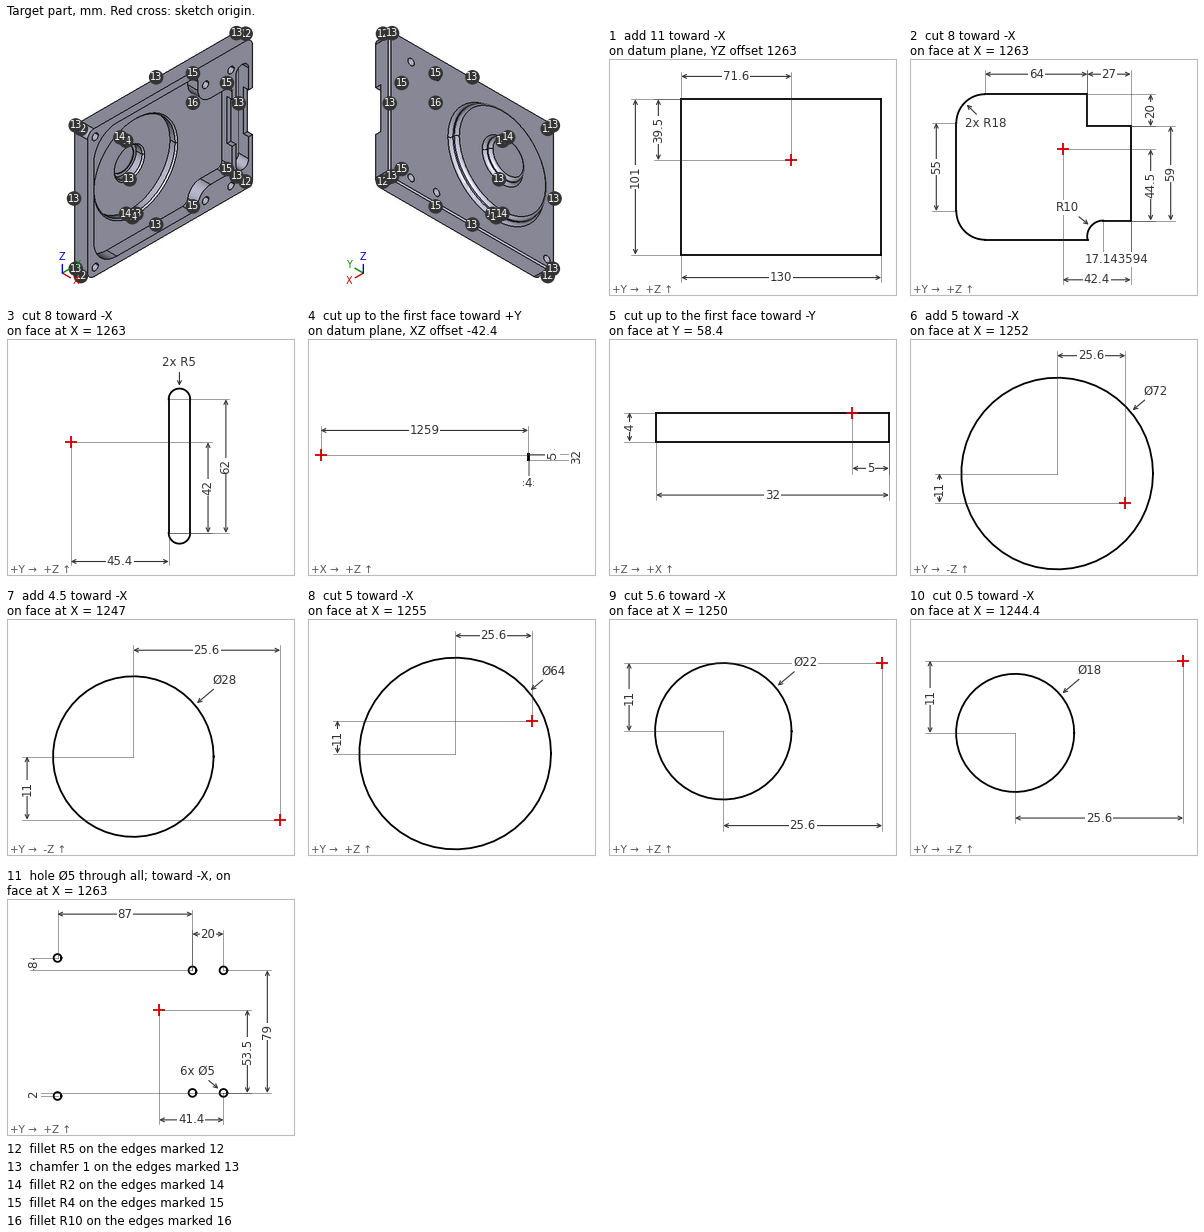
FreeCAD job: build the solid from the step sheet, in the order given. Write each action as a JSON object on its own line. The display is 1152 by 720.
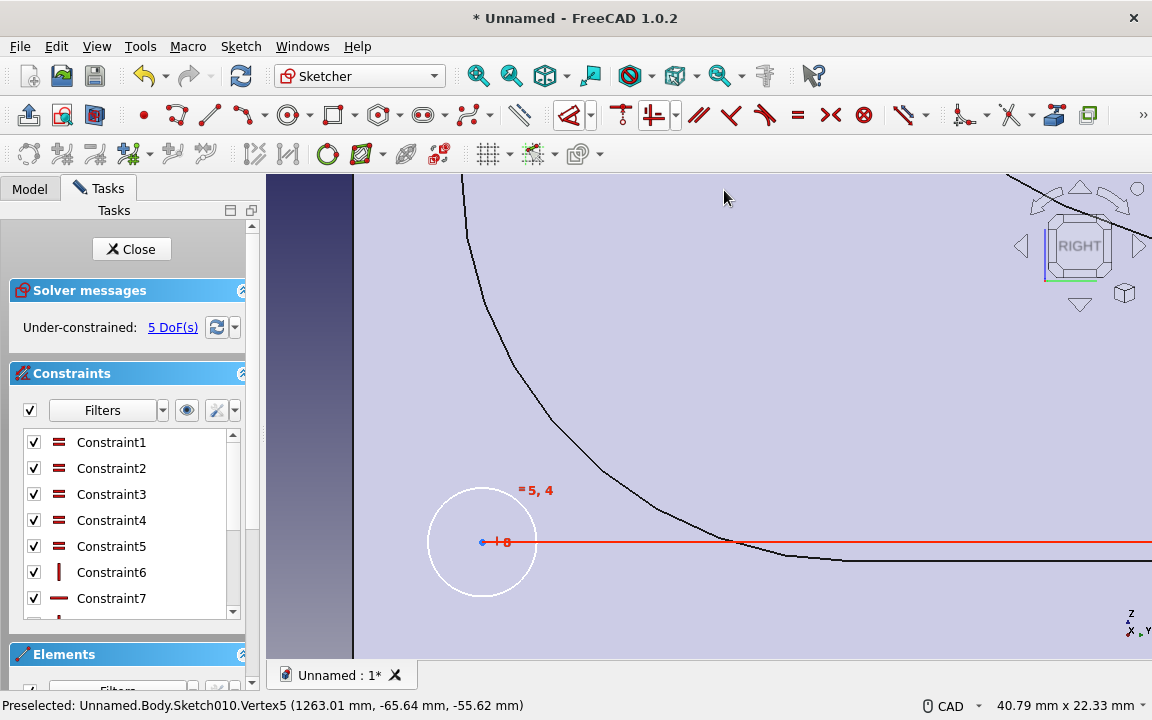
{"action": "scroll", "coordinate": [483, 549], "scroll_direction": "down", "scroll_amount": 10}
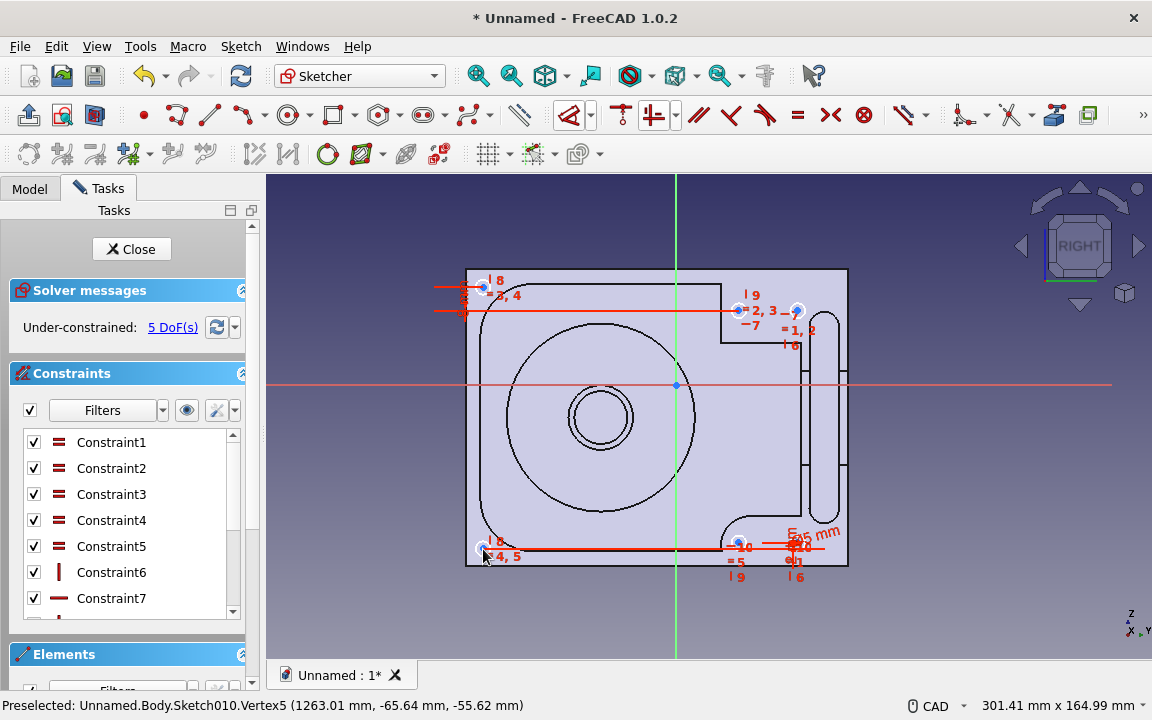
{"action": "left_click", "coordinate": [798, 543]}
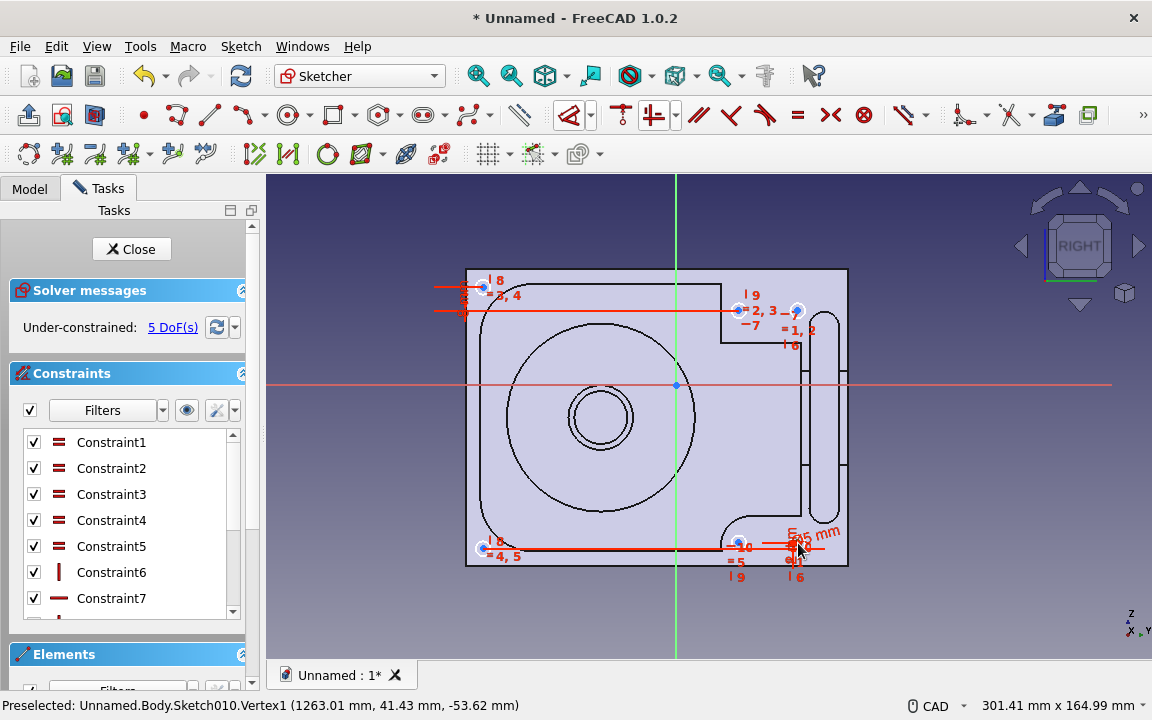
{"action": "left_click", "coordinate": [798, 311]}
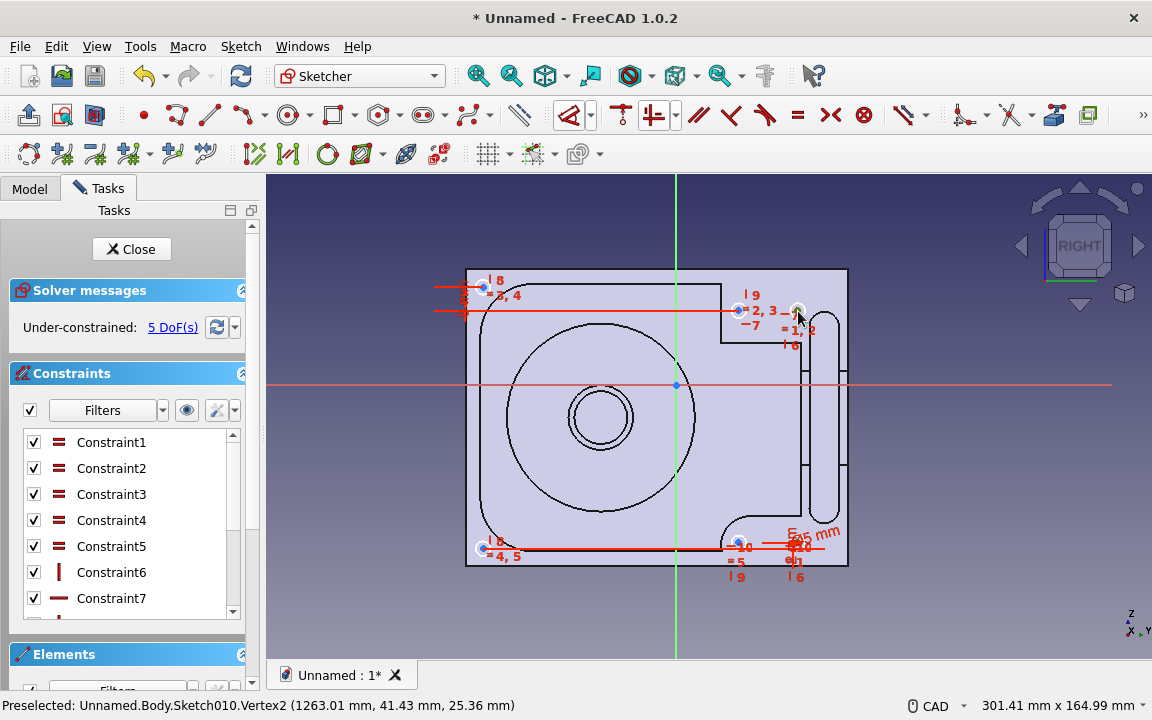
{"action": "key", "text": "i"}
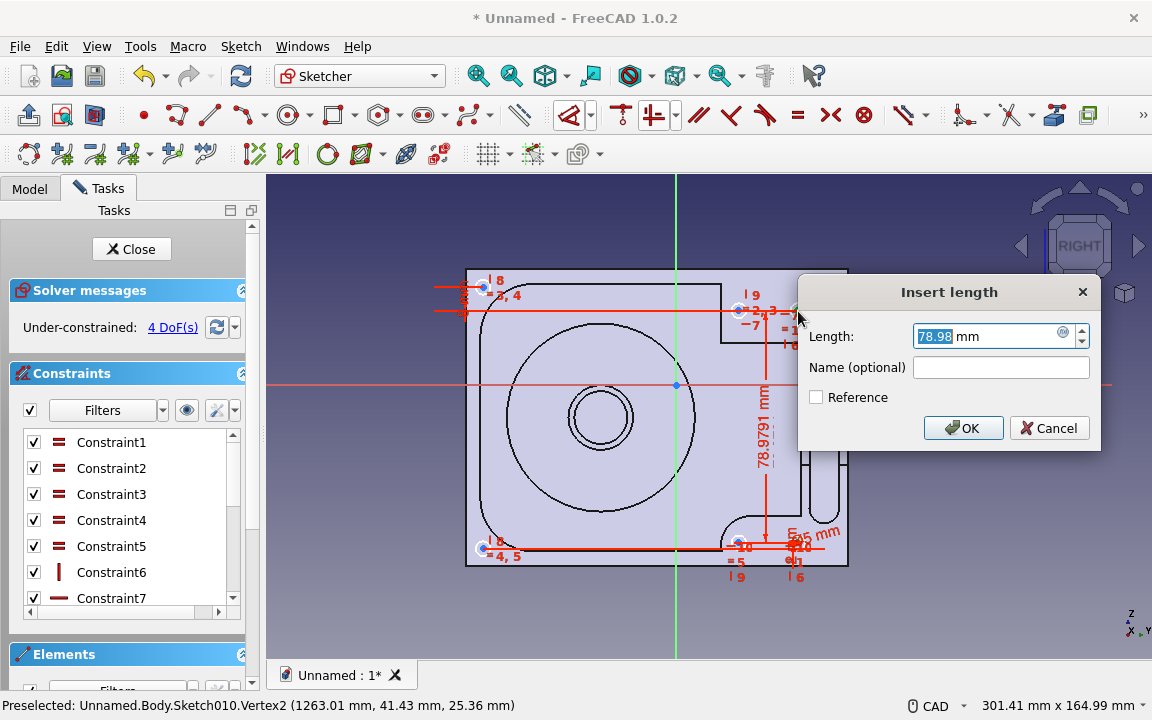
{"action": "type", "text": "79"}
{"action": "key", "text": "Return"}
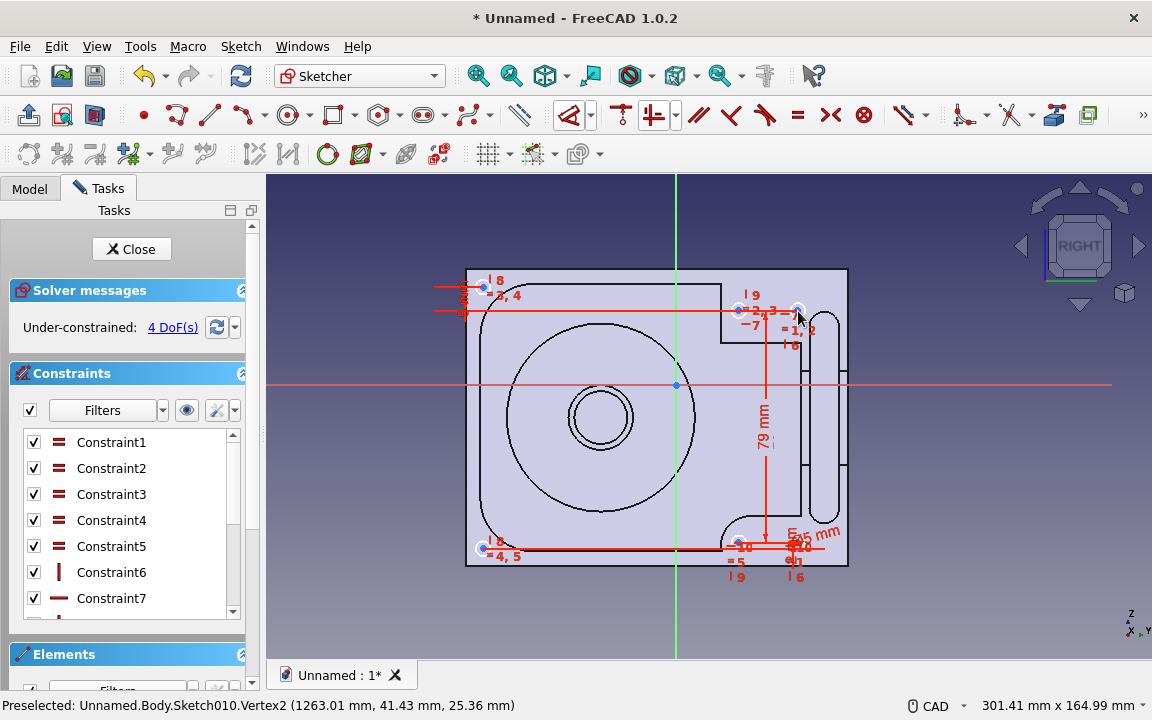
{"action": "left_click", "coordinate": [798, 311]}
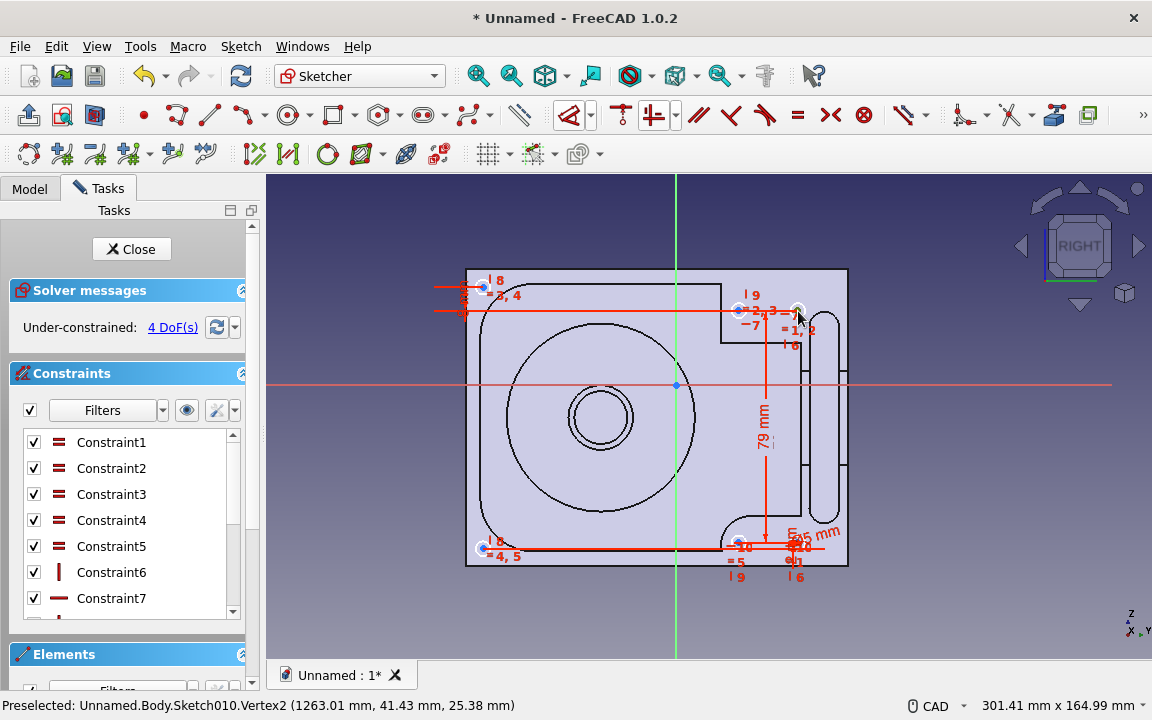
{"action": "left_click", "coordinate": [739, 311]}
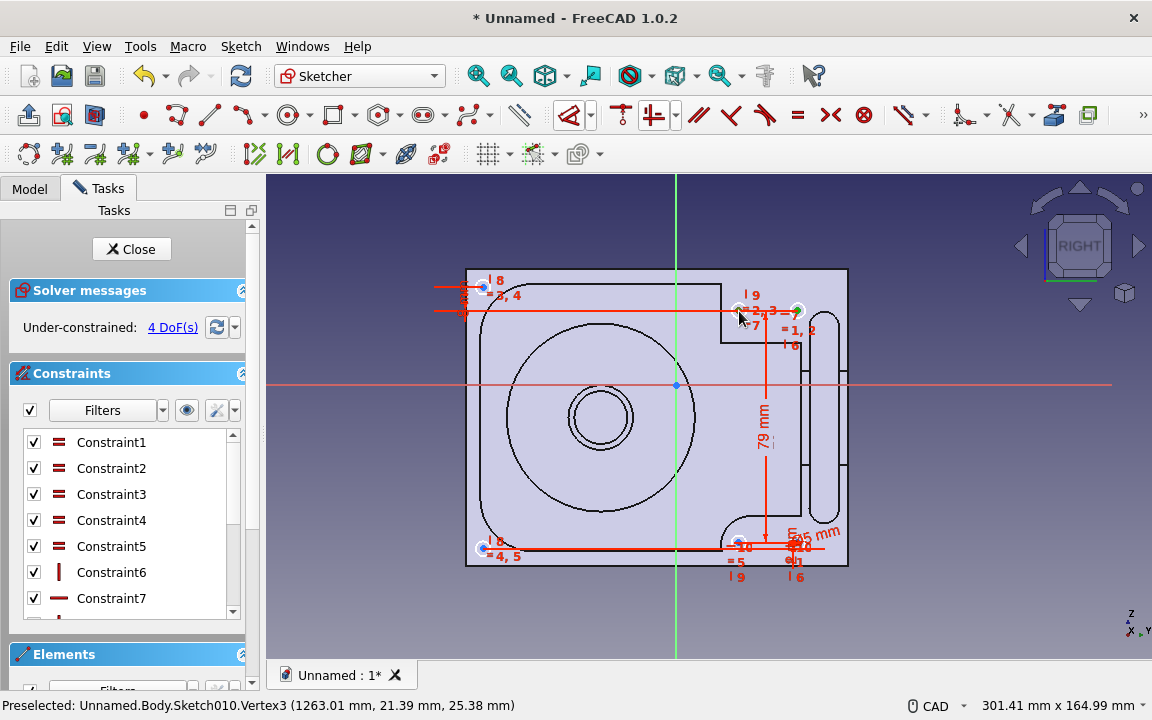
{"action": "left_click", "coordinate": [590, 116]}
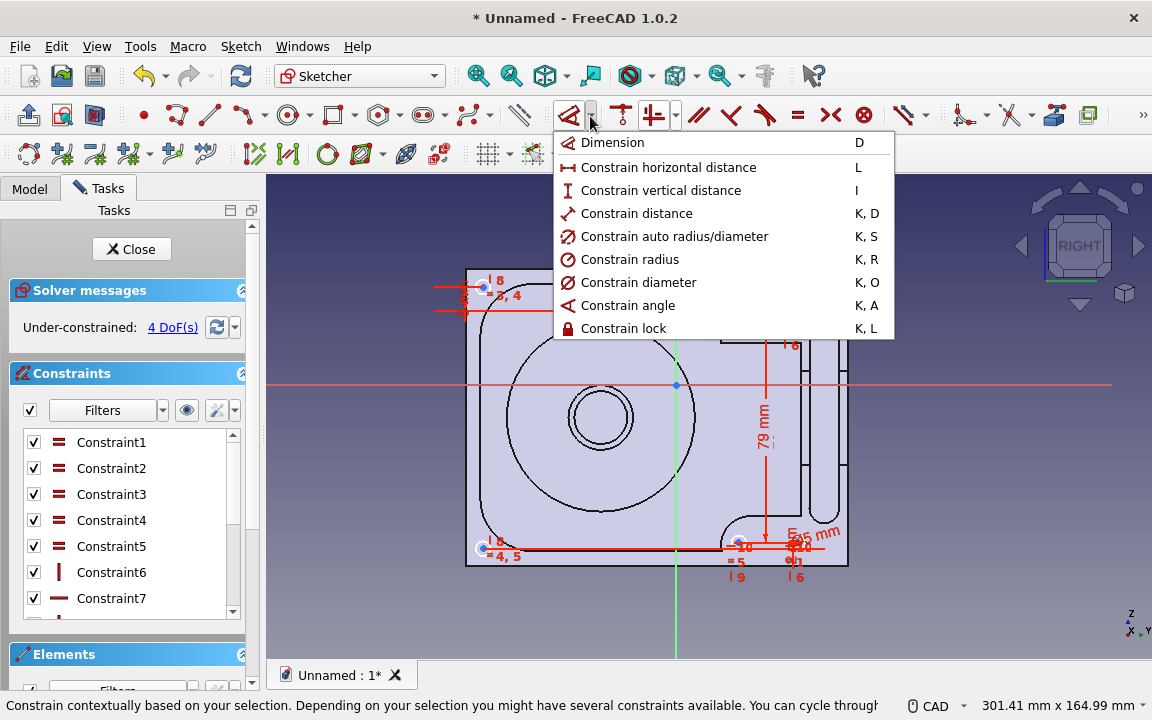
{"action": "left_click", "coordinate": [724, 168]}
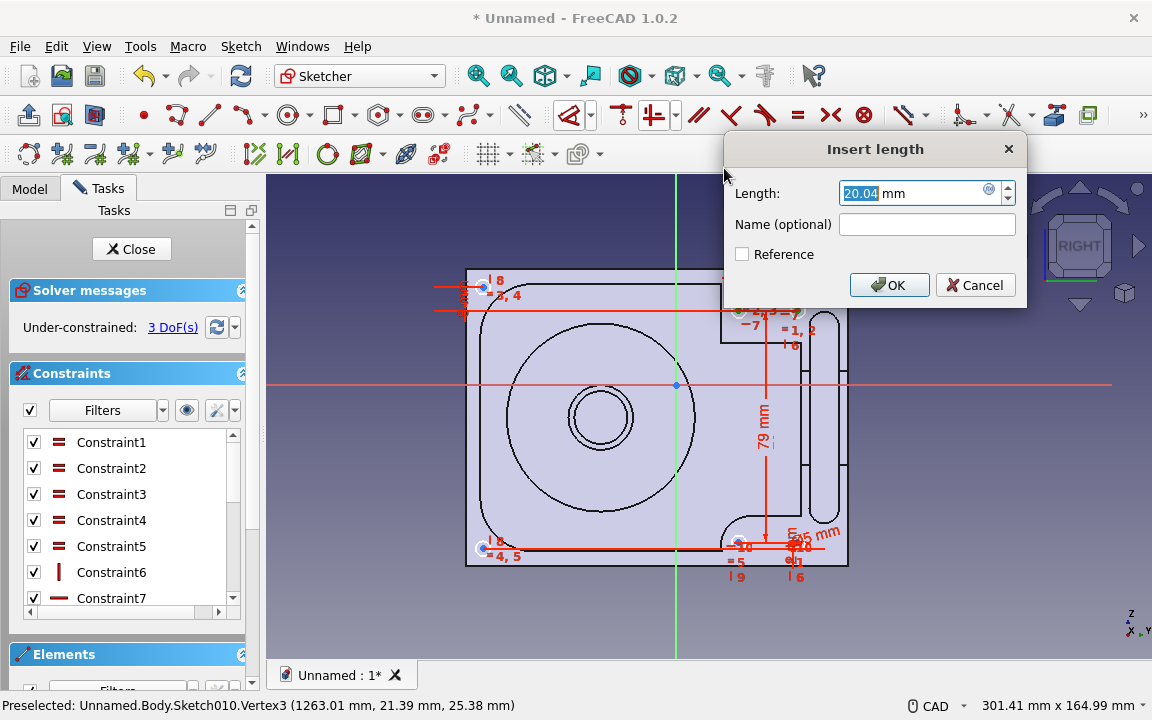
{"action": "type", "text": "20"}
{"action": "key", "text": "Return"}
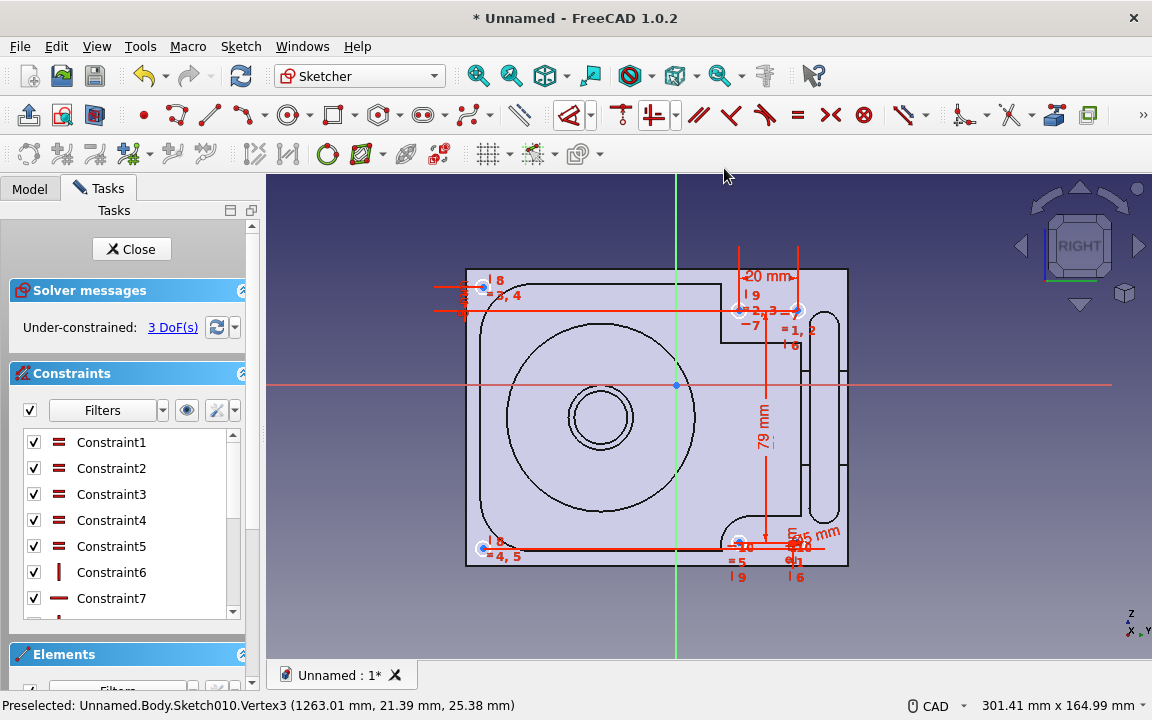
{"action": "left_click", "coordinate": [739, 311]}